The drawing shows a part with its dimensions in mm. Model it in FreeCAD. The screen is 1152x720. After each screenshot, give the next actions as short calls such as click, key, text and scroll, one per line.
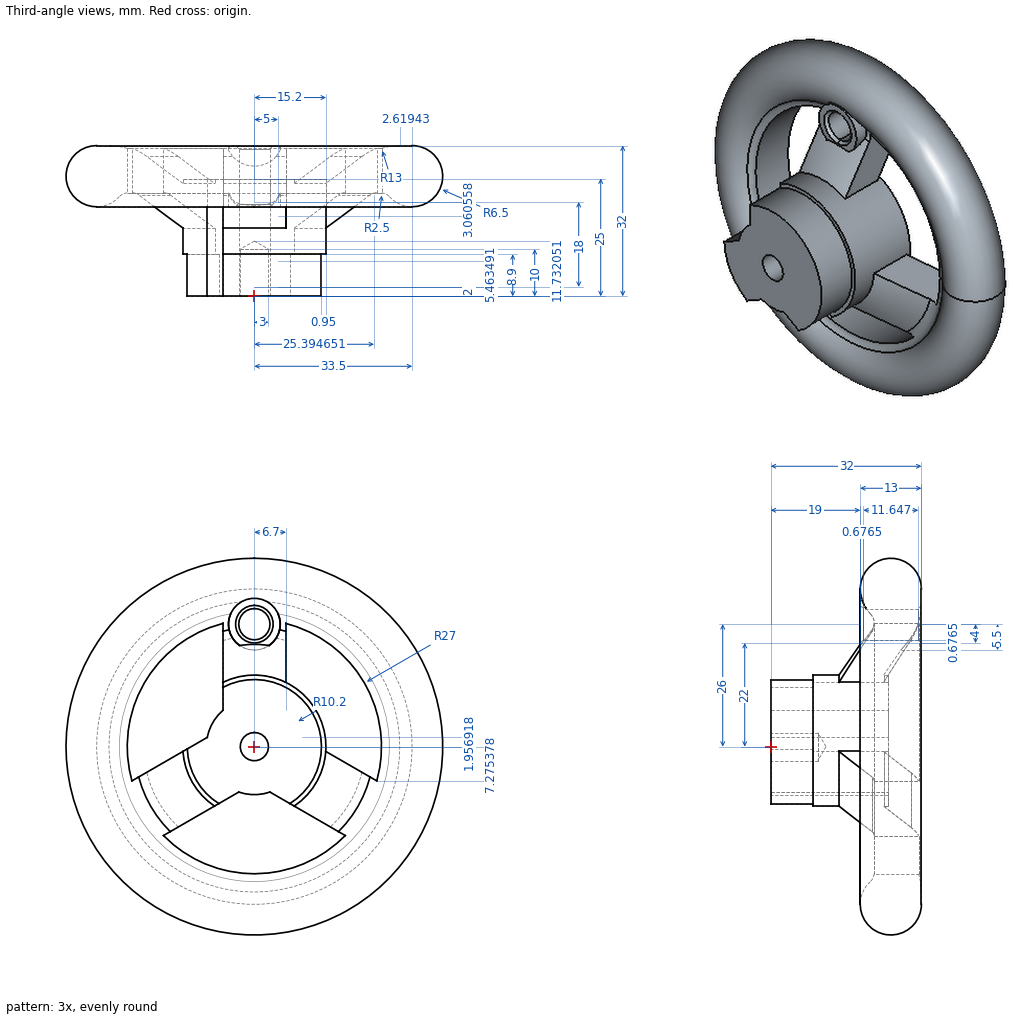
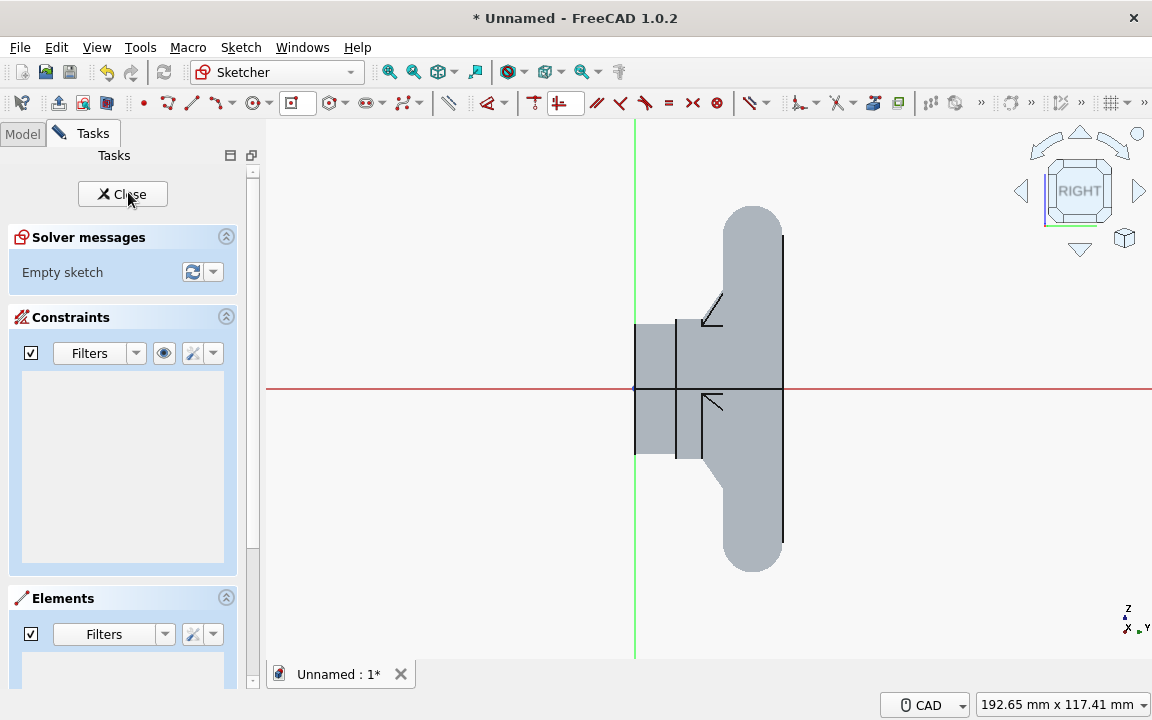
click(108, 104)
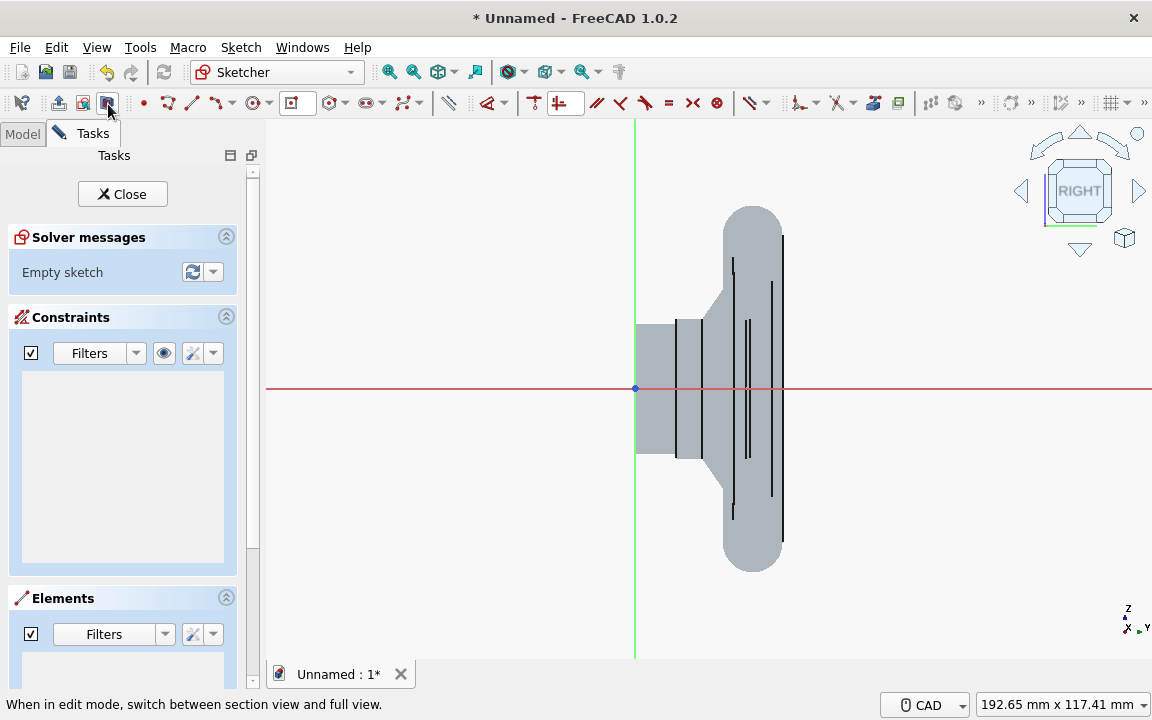
scroll(768, 294, up, 5)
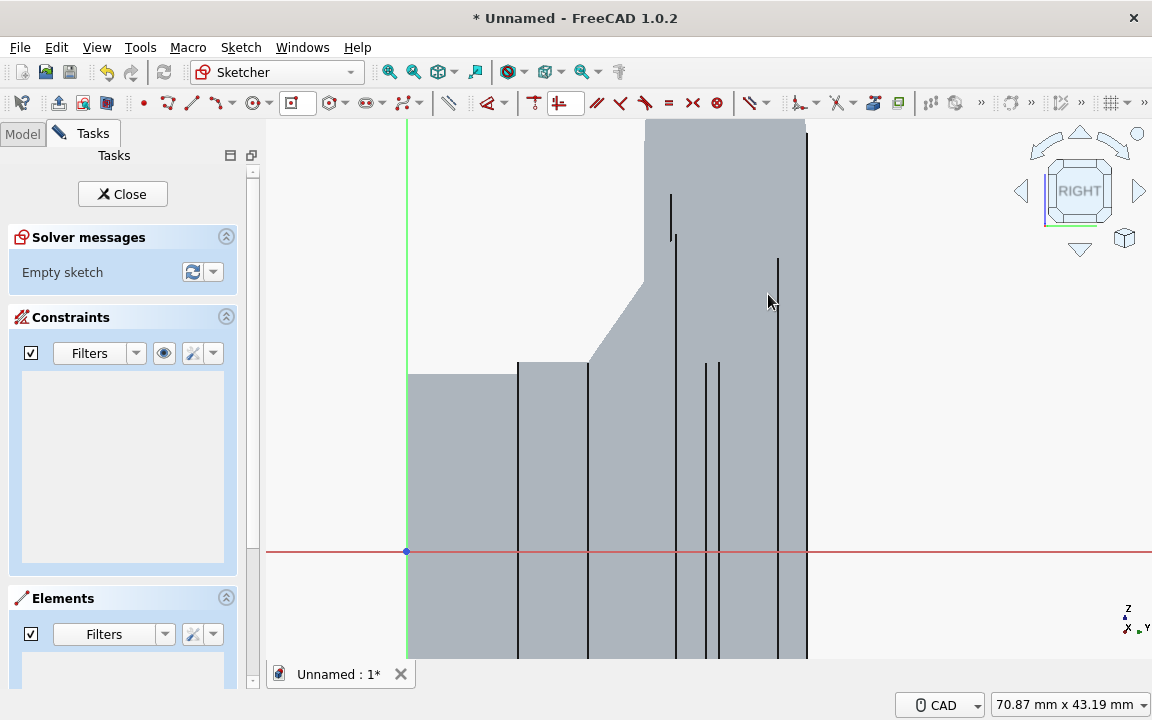
key(g)
key(r)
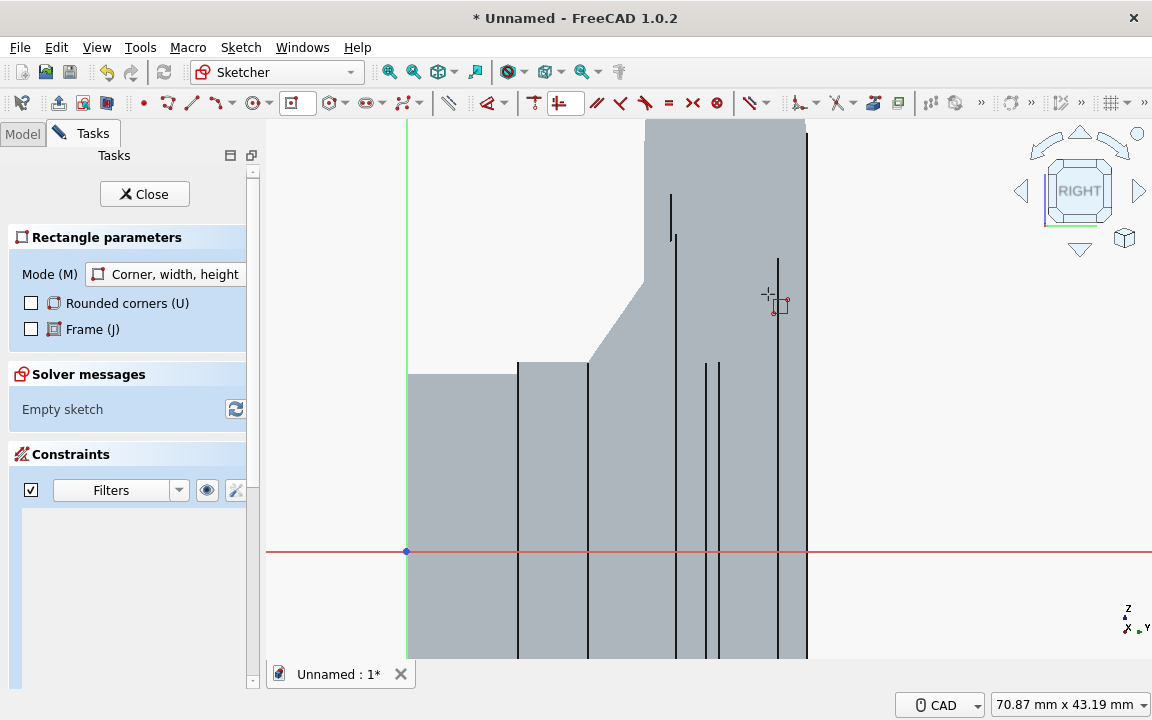
click(644, 227)
move(807, 295)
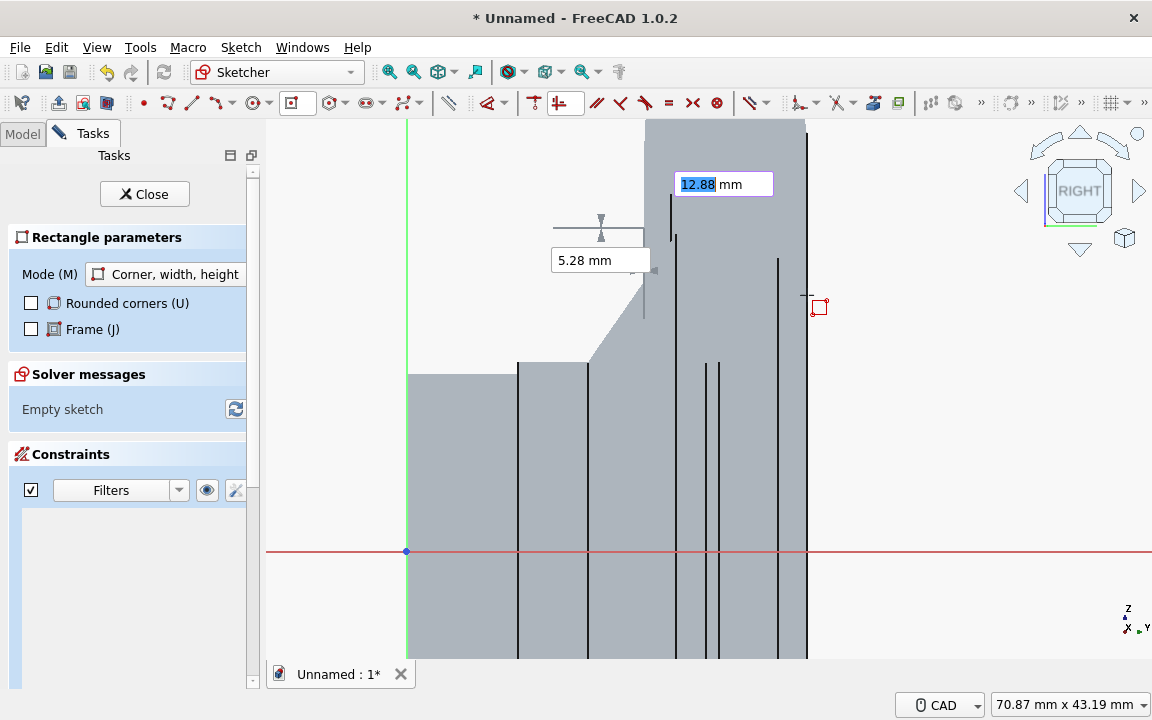
text(13)
key(Tab)
text(5.5)
key(Return)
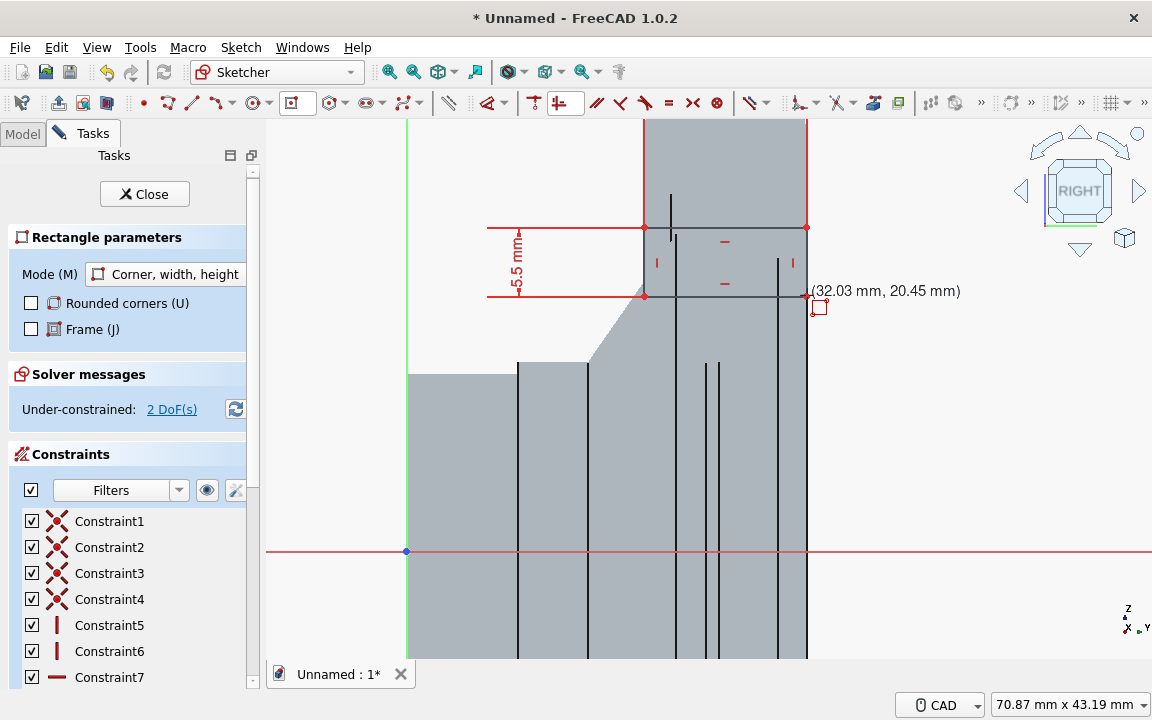
click(192, 104)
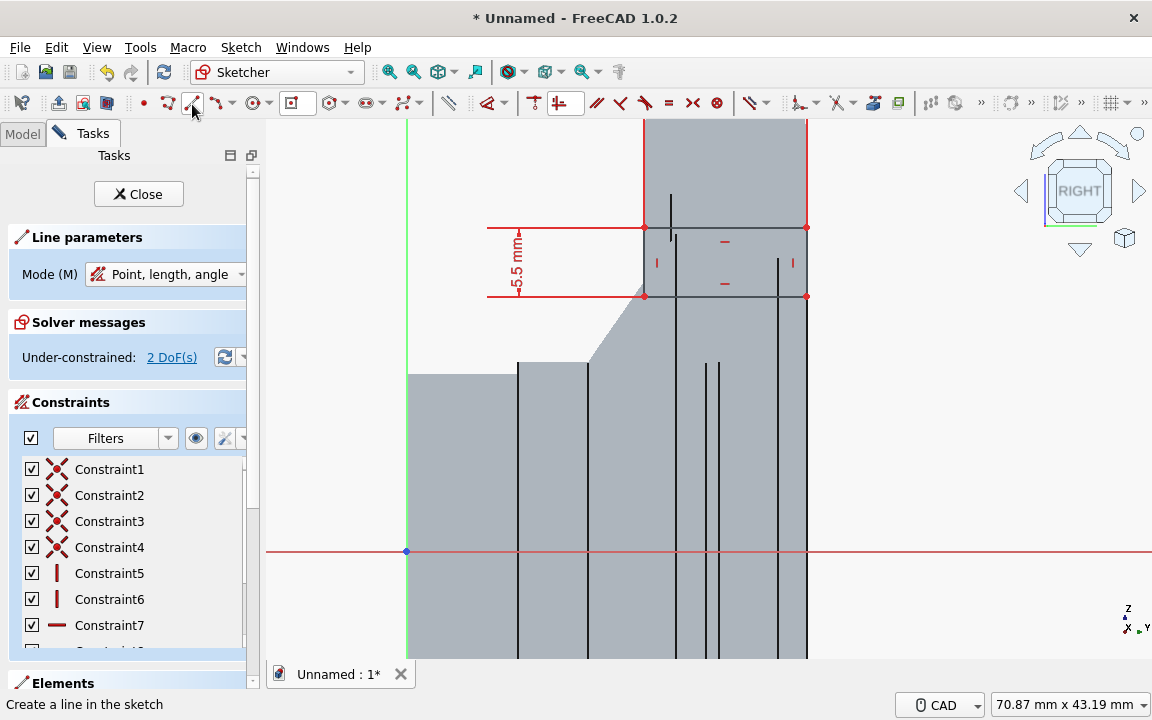
click(823, 227)
click(872, 227)
key(Escape)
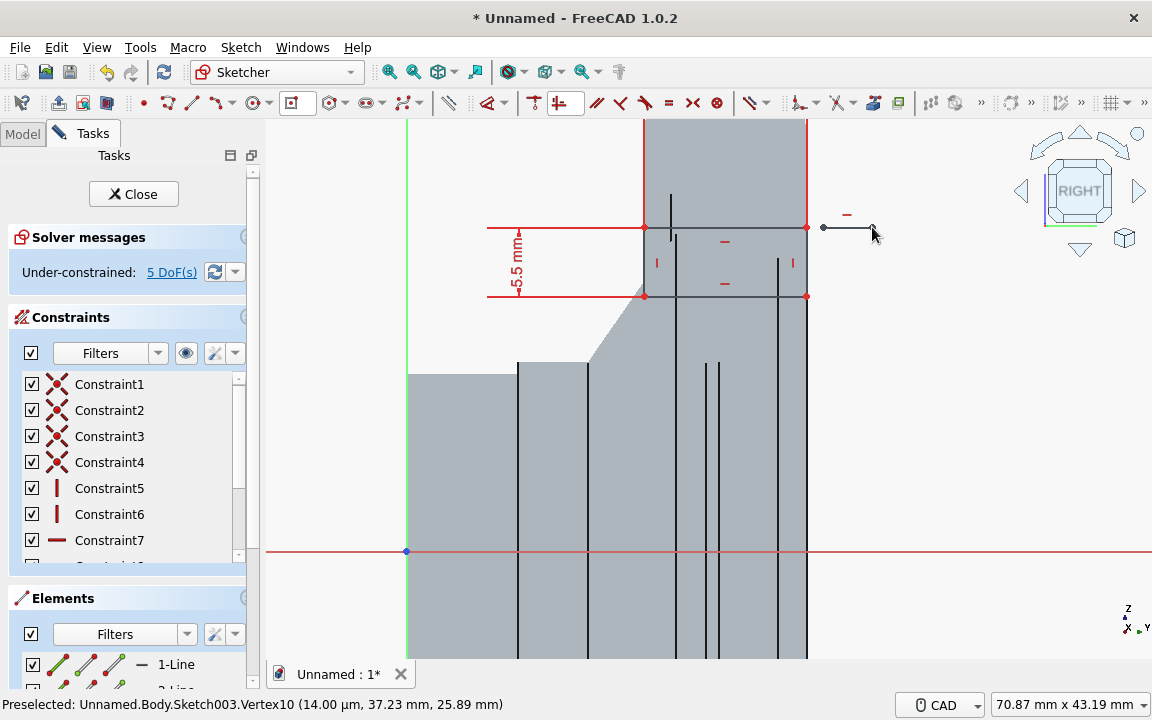
click(838, 228)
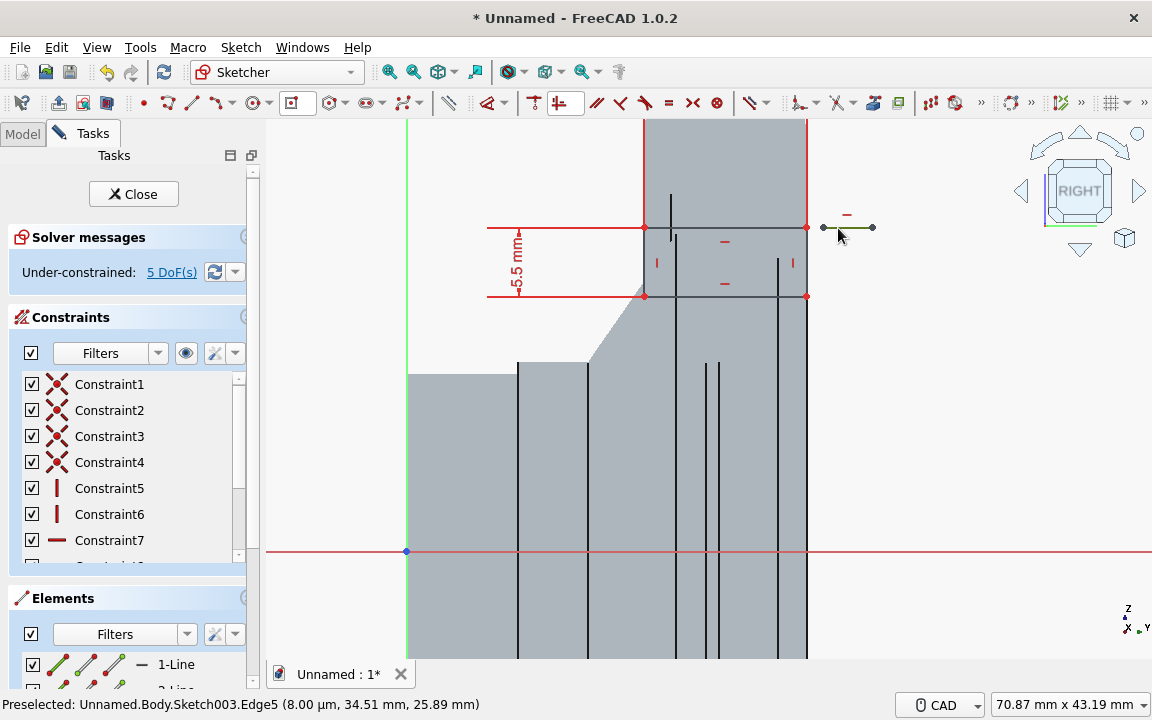
click(450, 104)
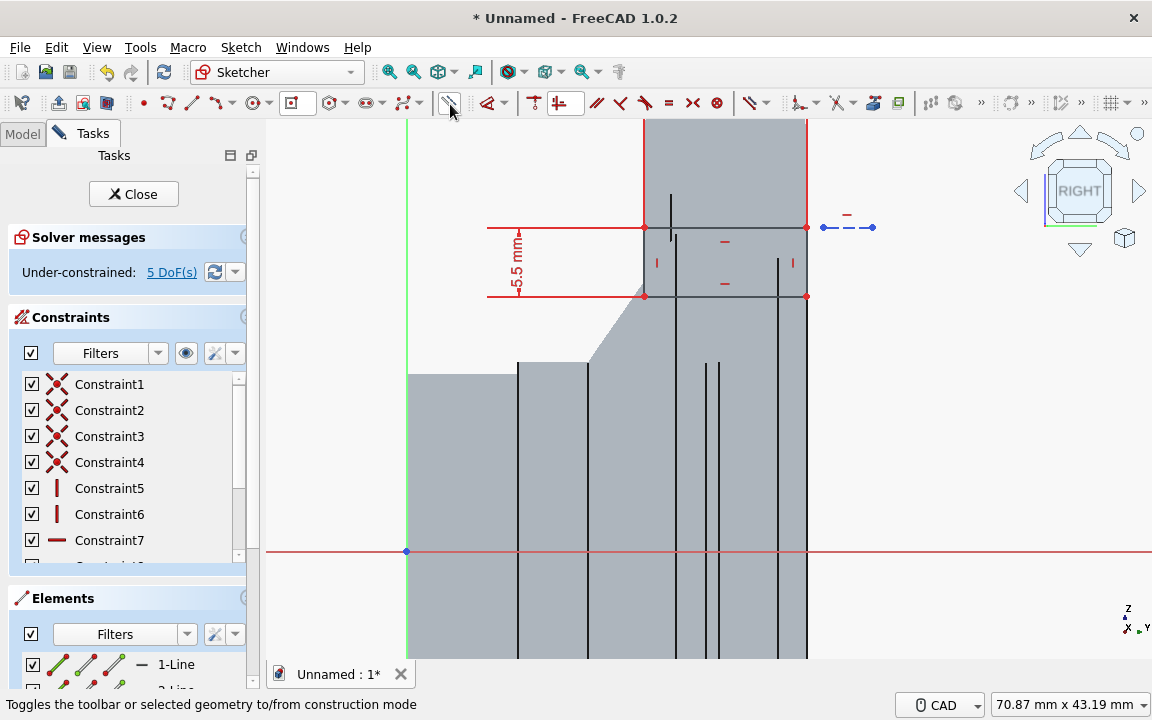
click(488, 104)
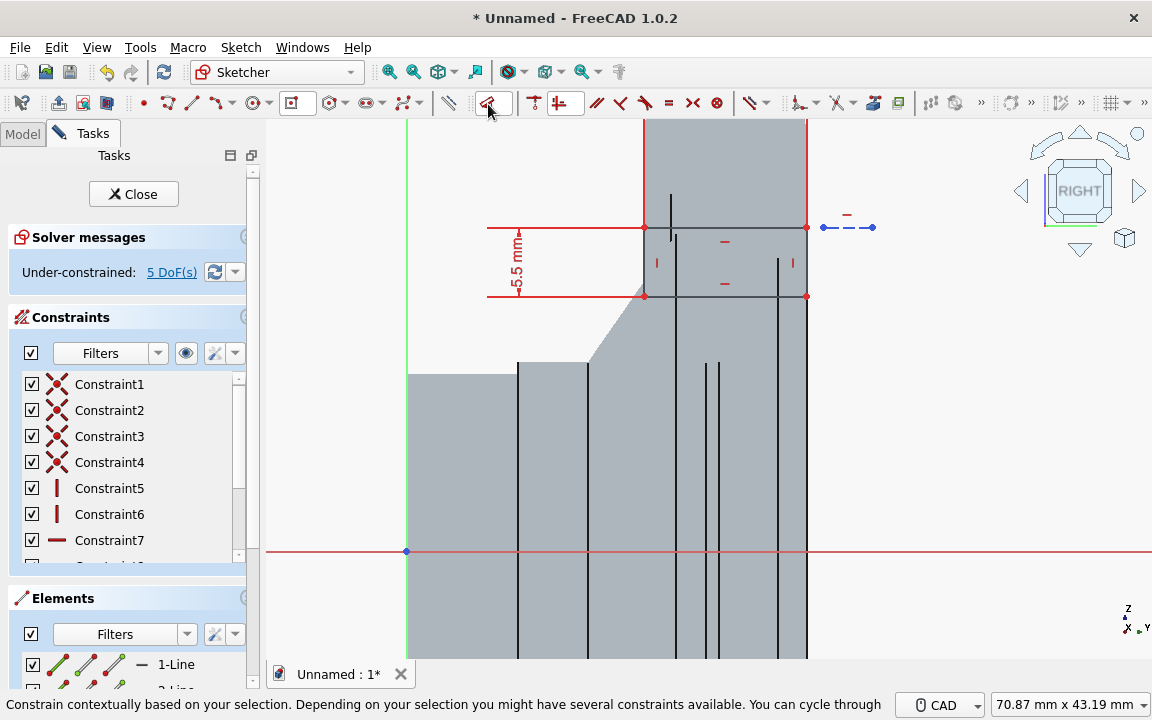
click(644, 228)
click(525, 586)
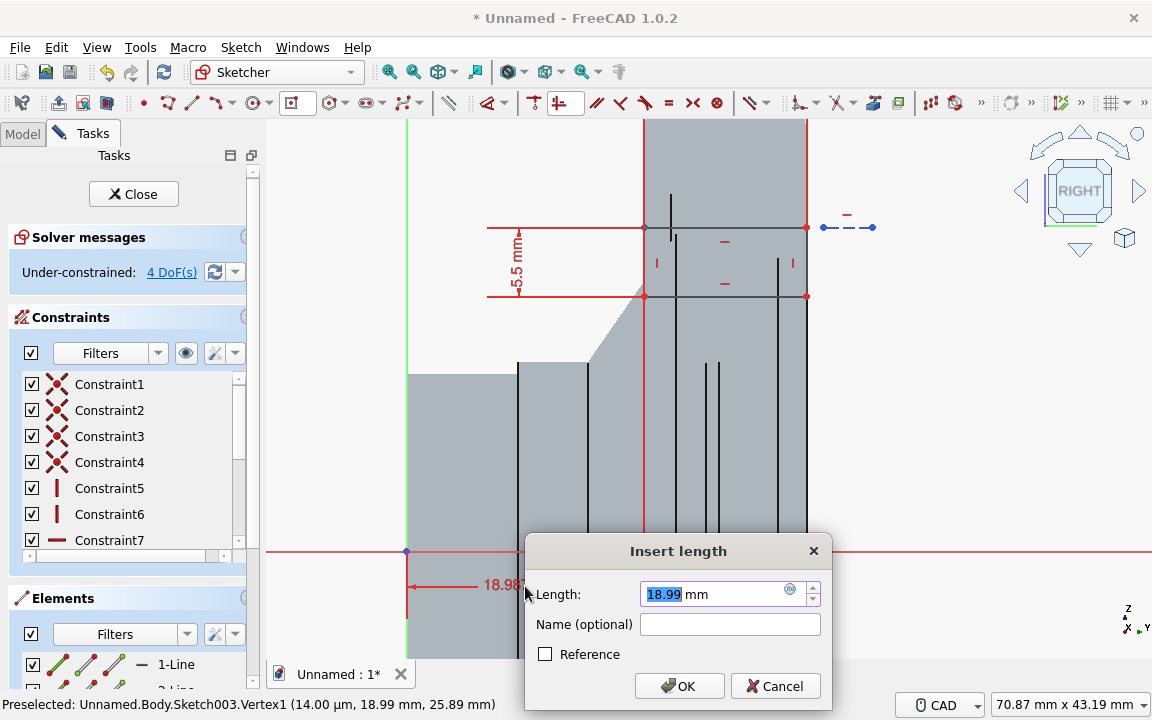
text(19)
key(Return)